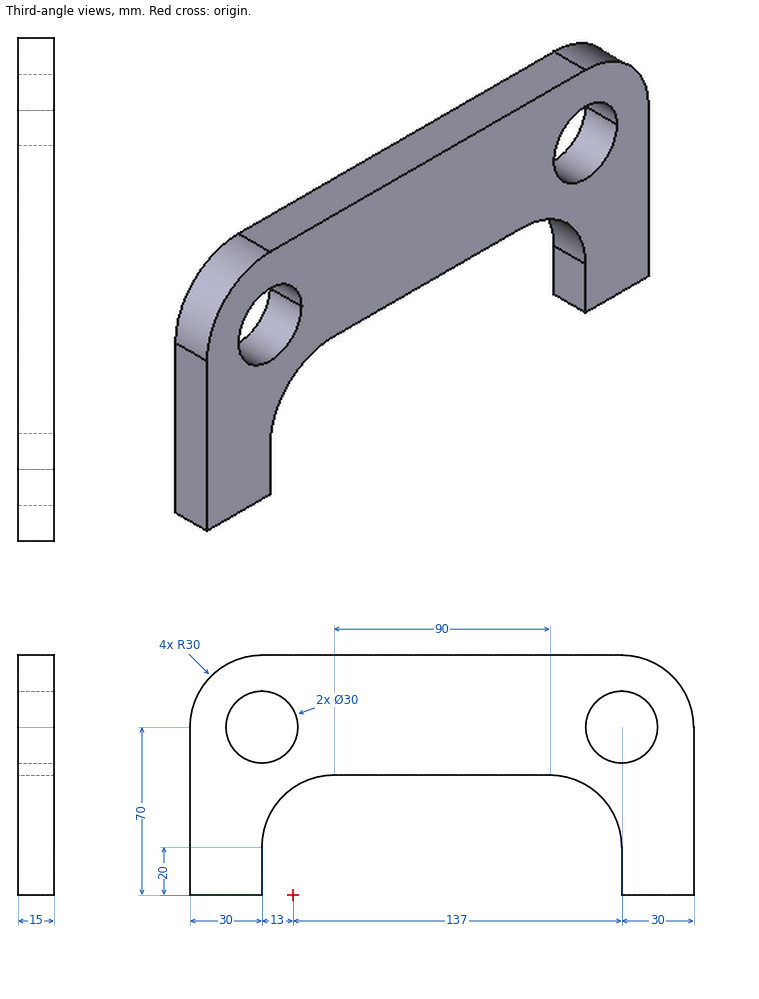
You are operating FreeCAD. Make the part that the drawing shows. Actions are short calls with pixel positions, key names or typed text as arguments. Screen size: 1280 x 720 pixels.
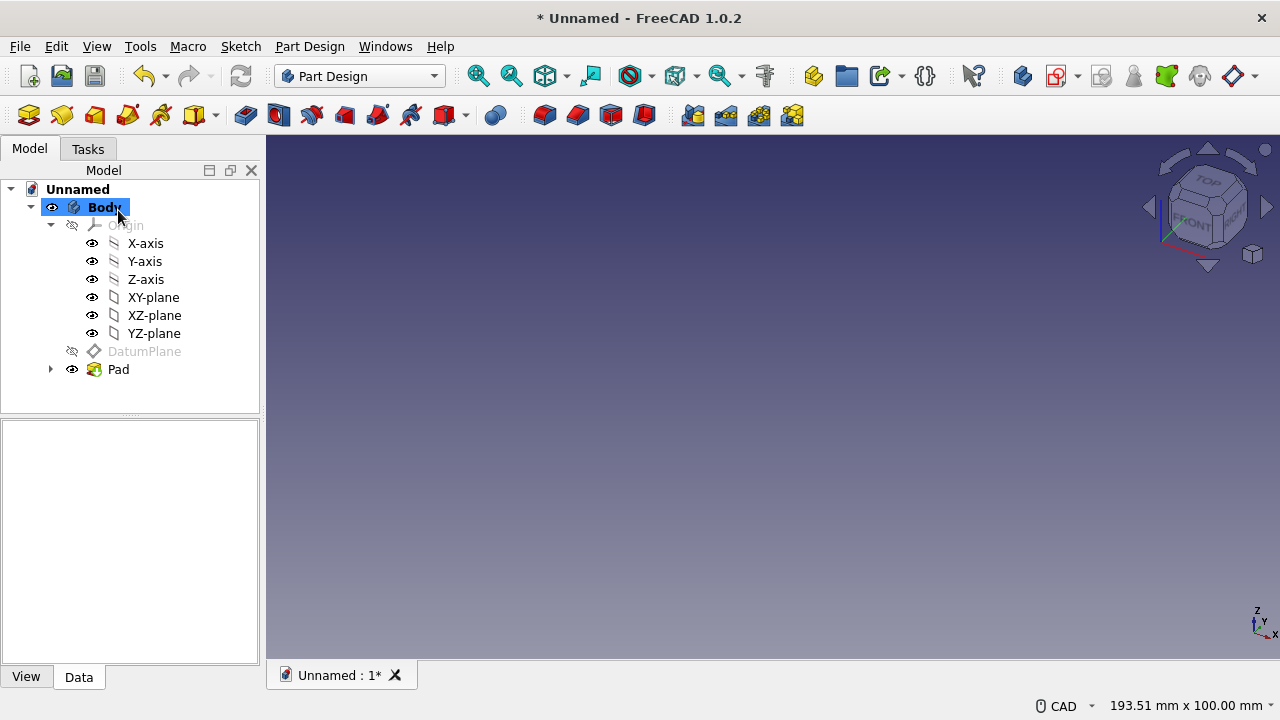
key(v)
key(f)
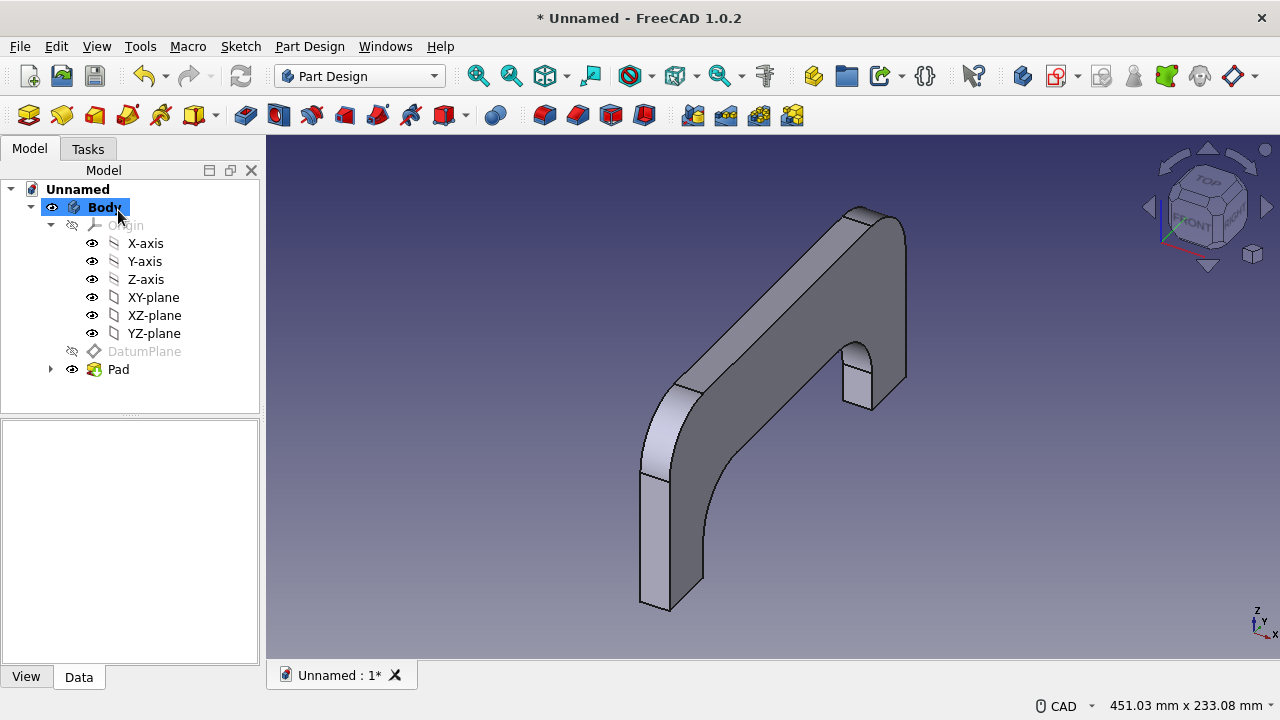
key(6)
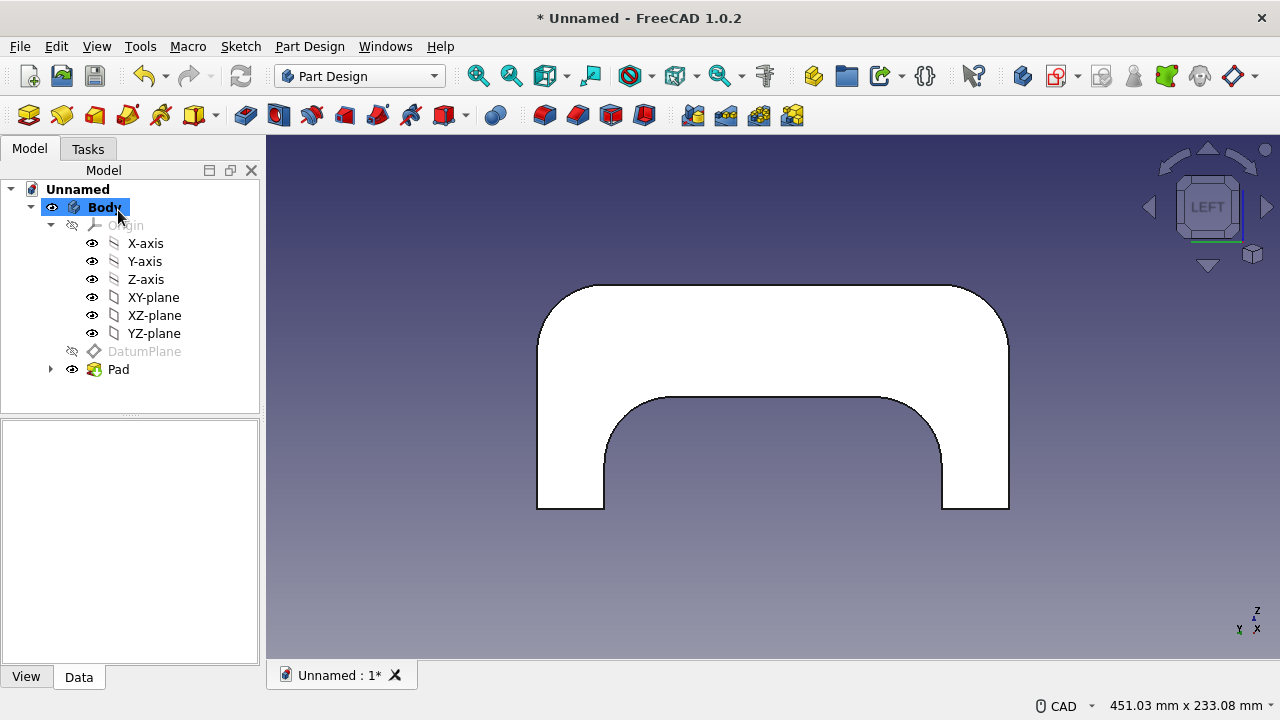
click(638, 332)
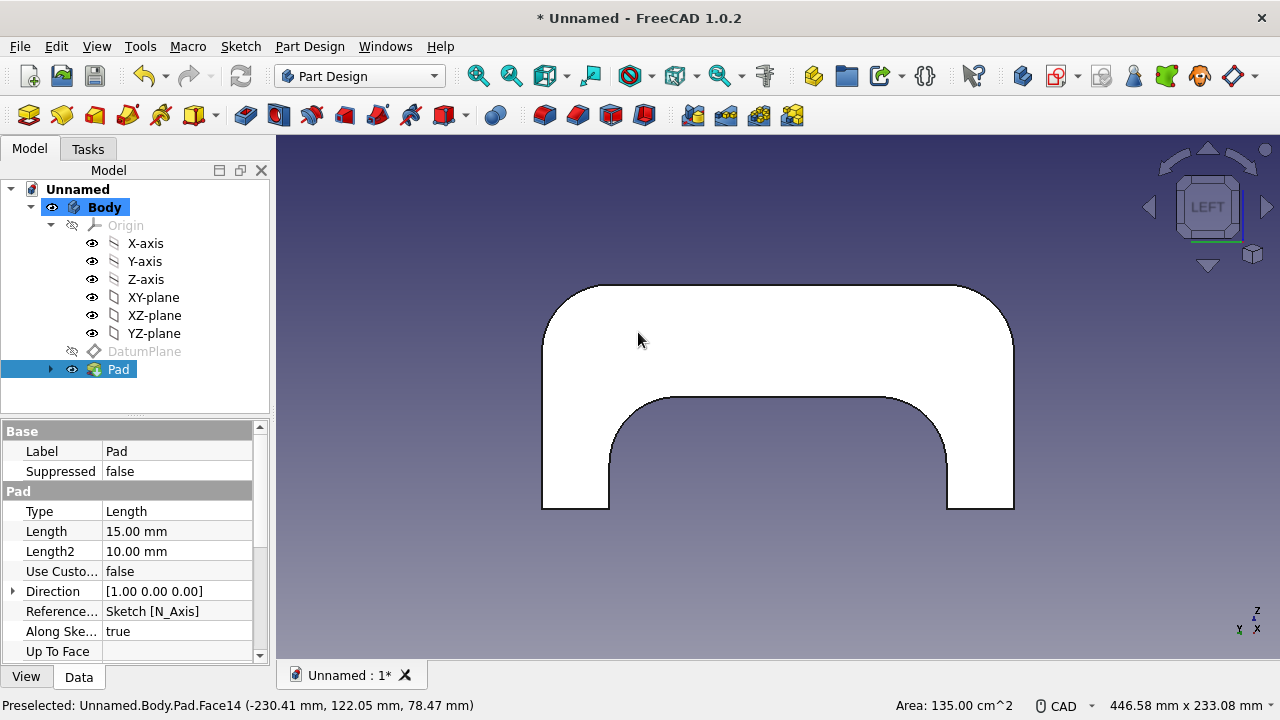
click(1056, 76)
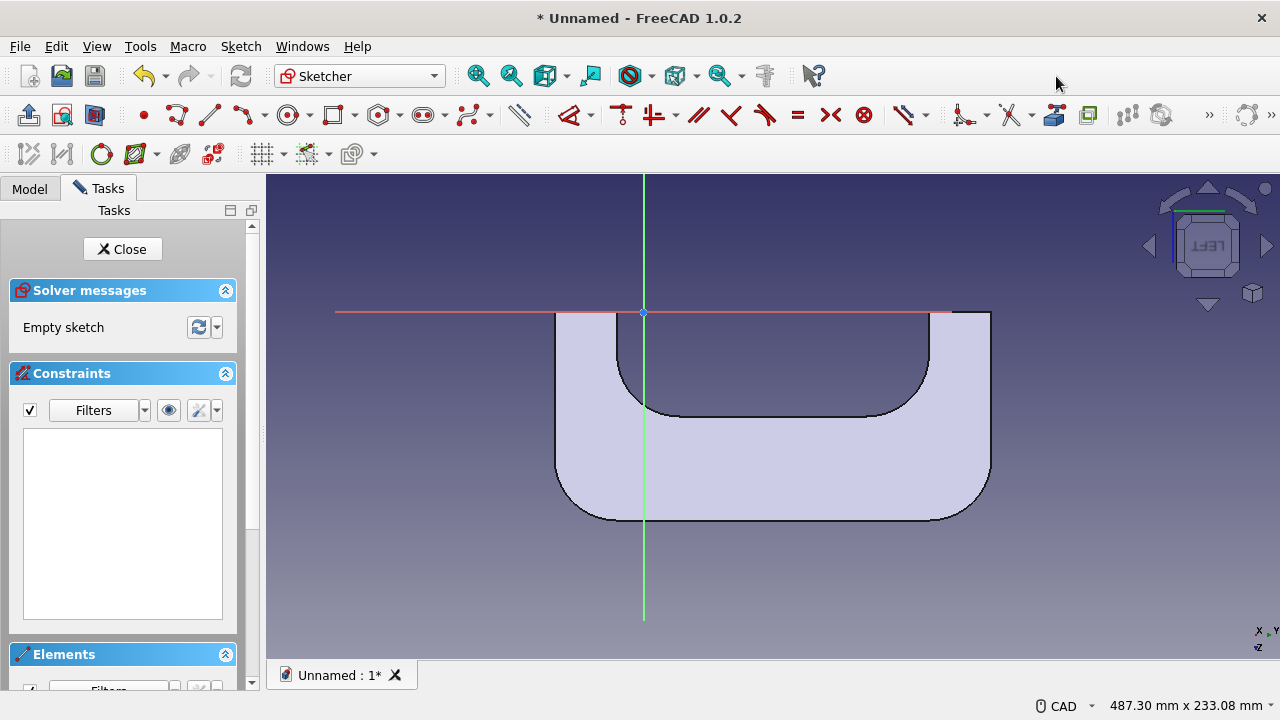
scroll(912, 369, up, 2)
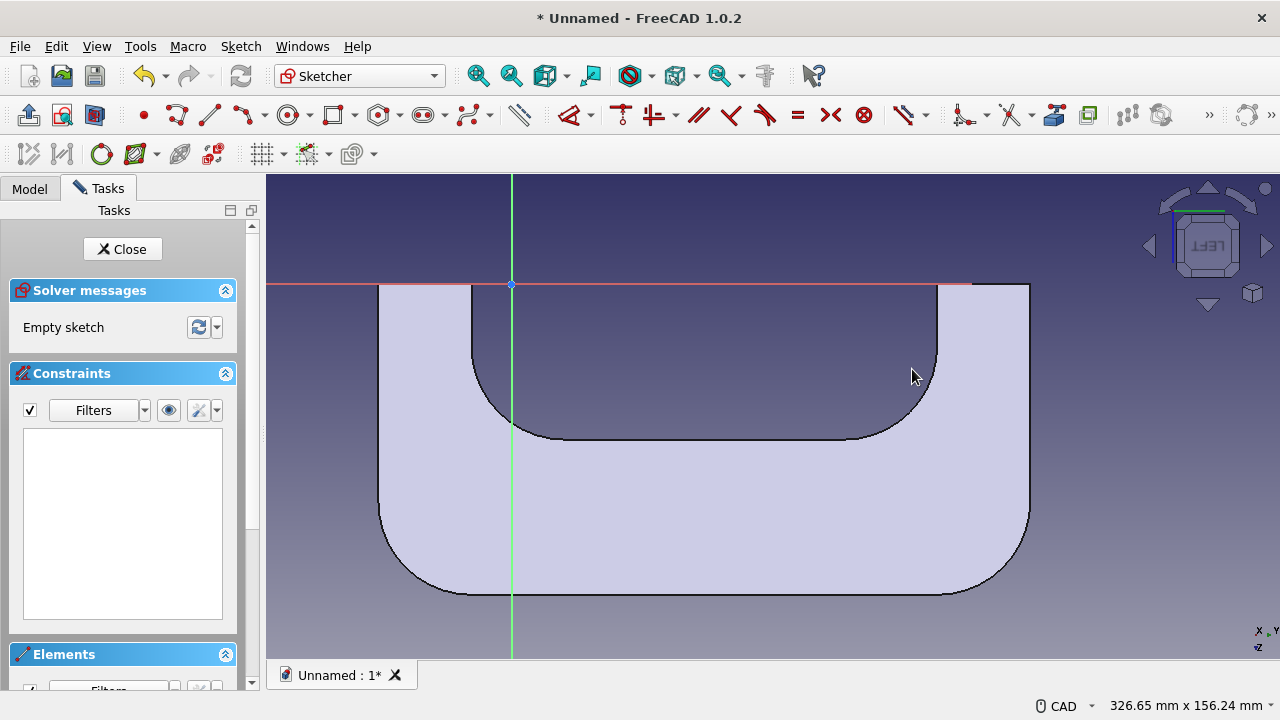
key(g)
key(c)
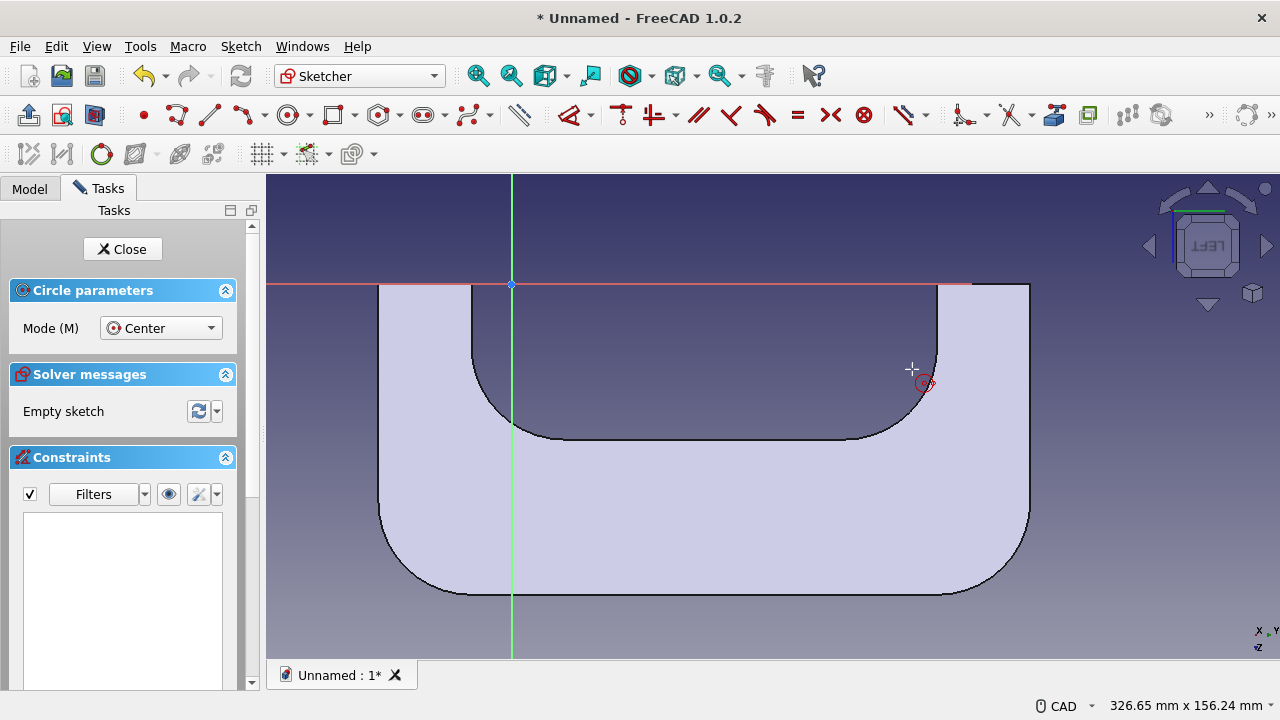
click(472, 502)
click(439, 469)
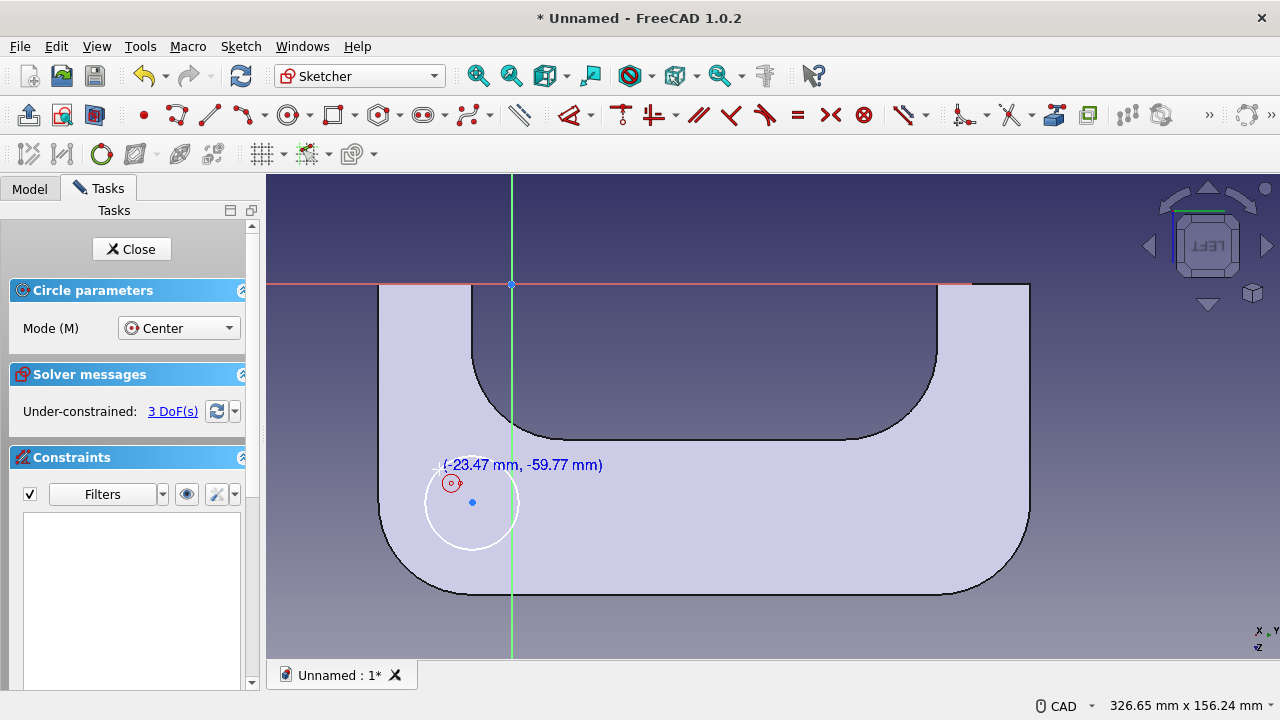
click(937, 502)
click(970, 469)
key(Escape)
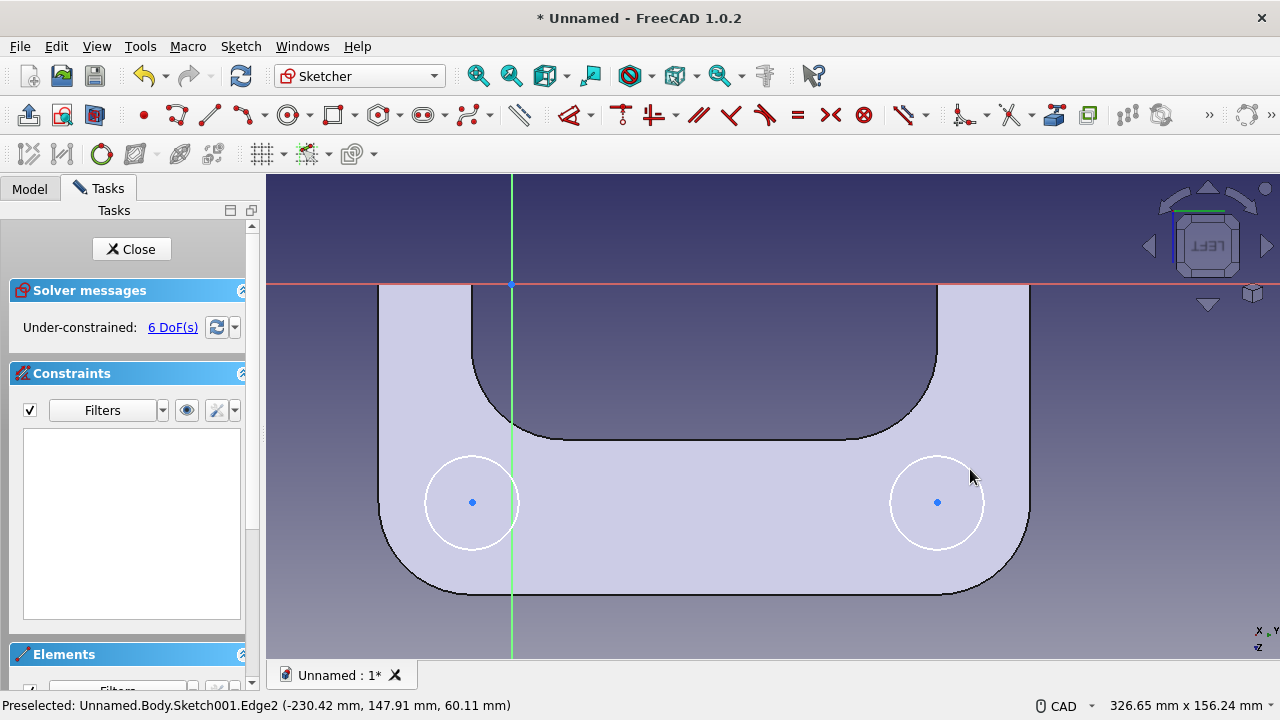
click(439, 470)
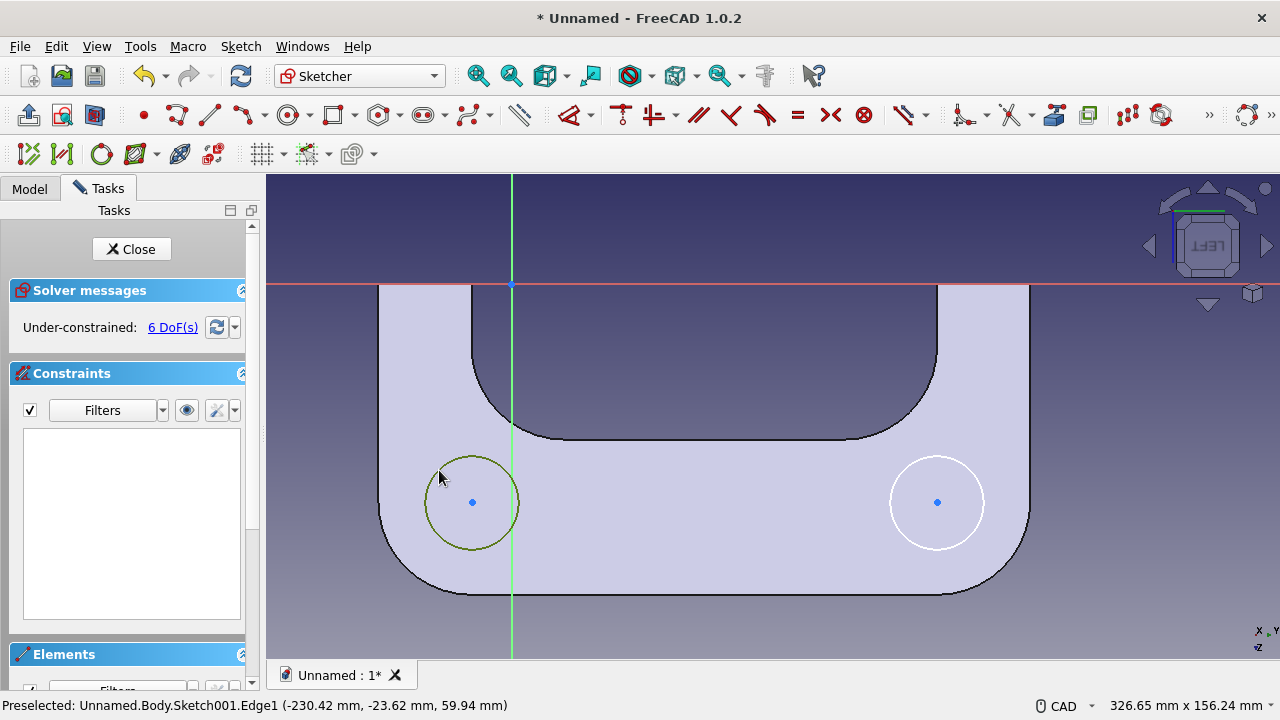
click(970, 470)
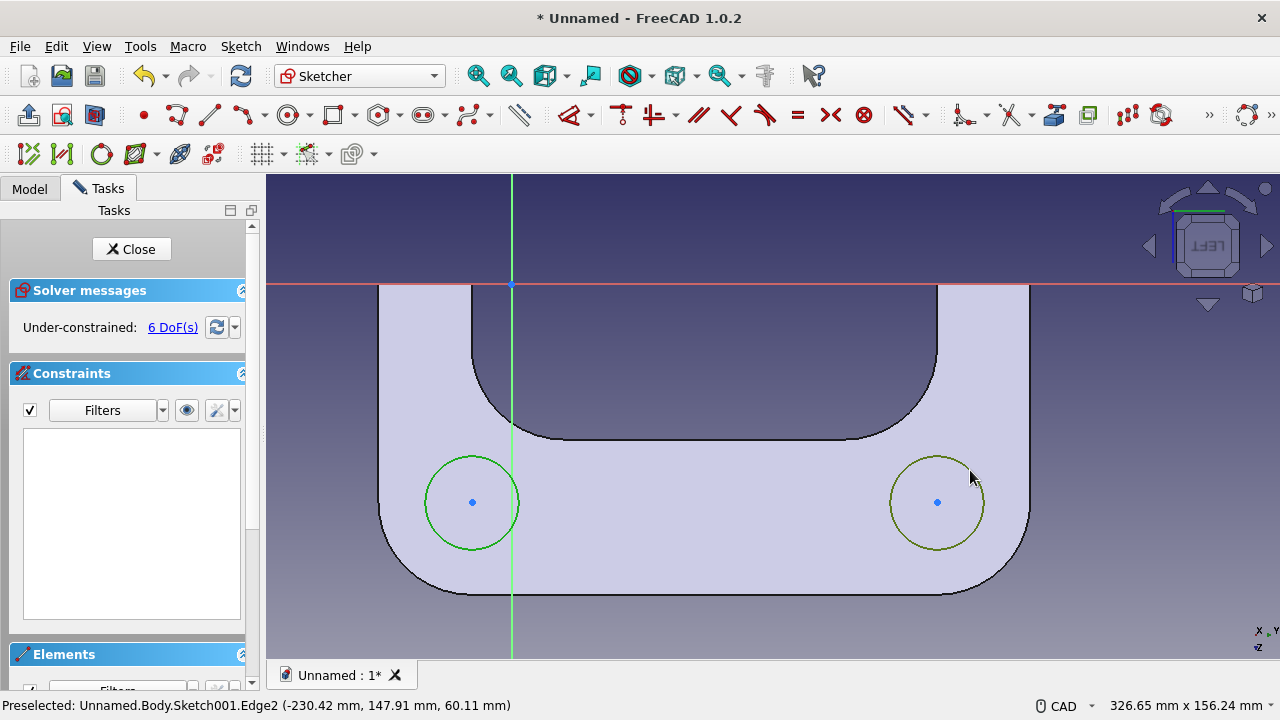
key(e)